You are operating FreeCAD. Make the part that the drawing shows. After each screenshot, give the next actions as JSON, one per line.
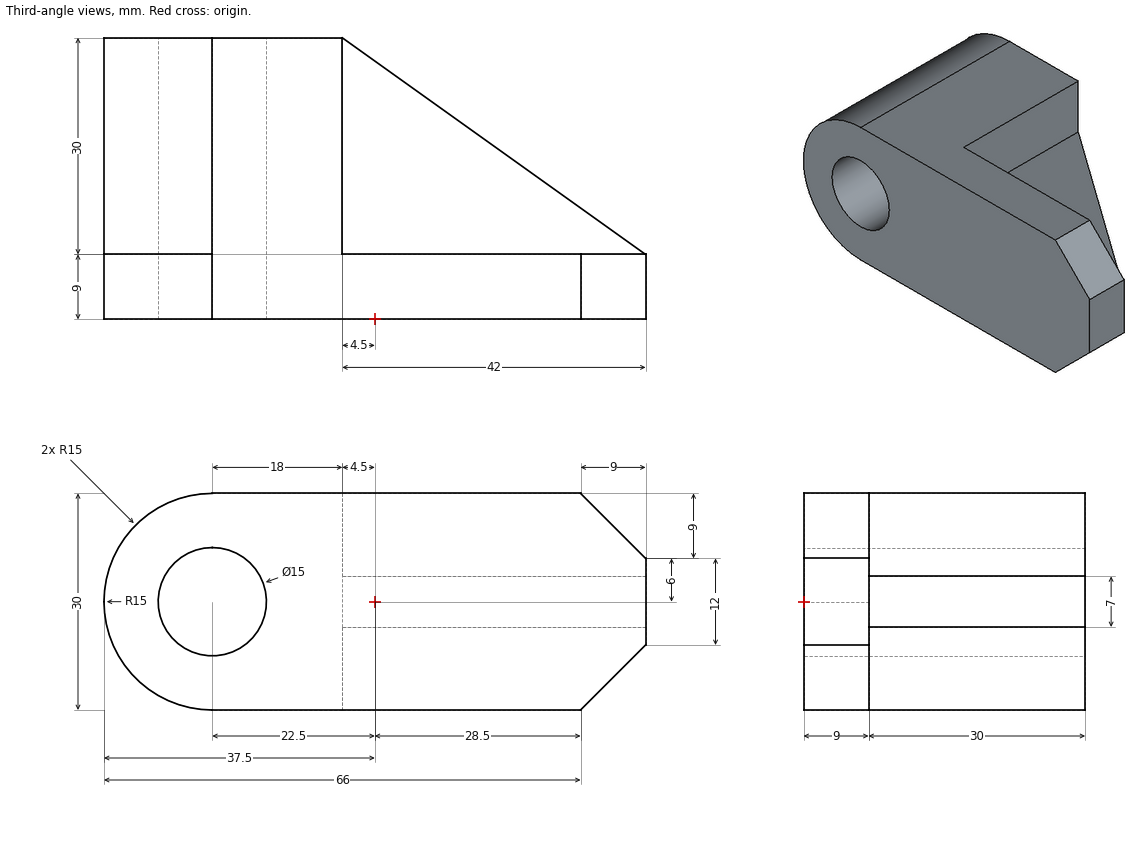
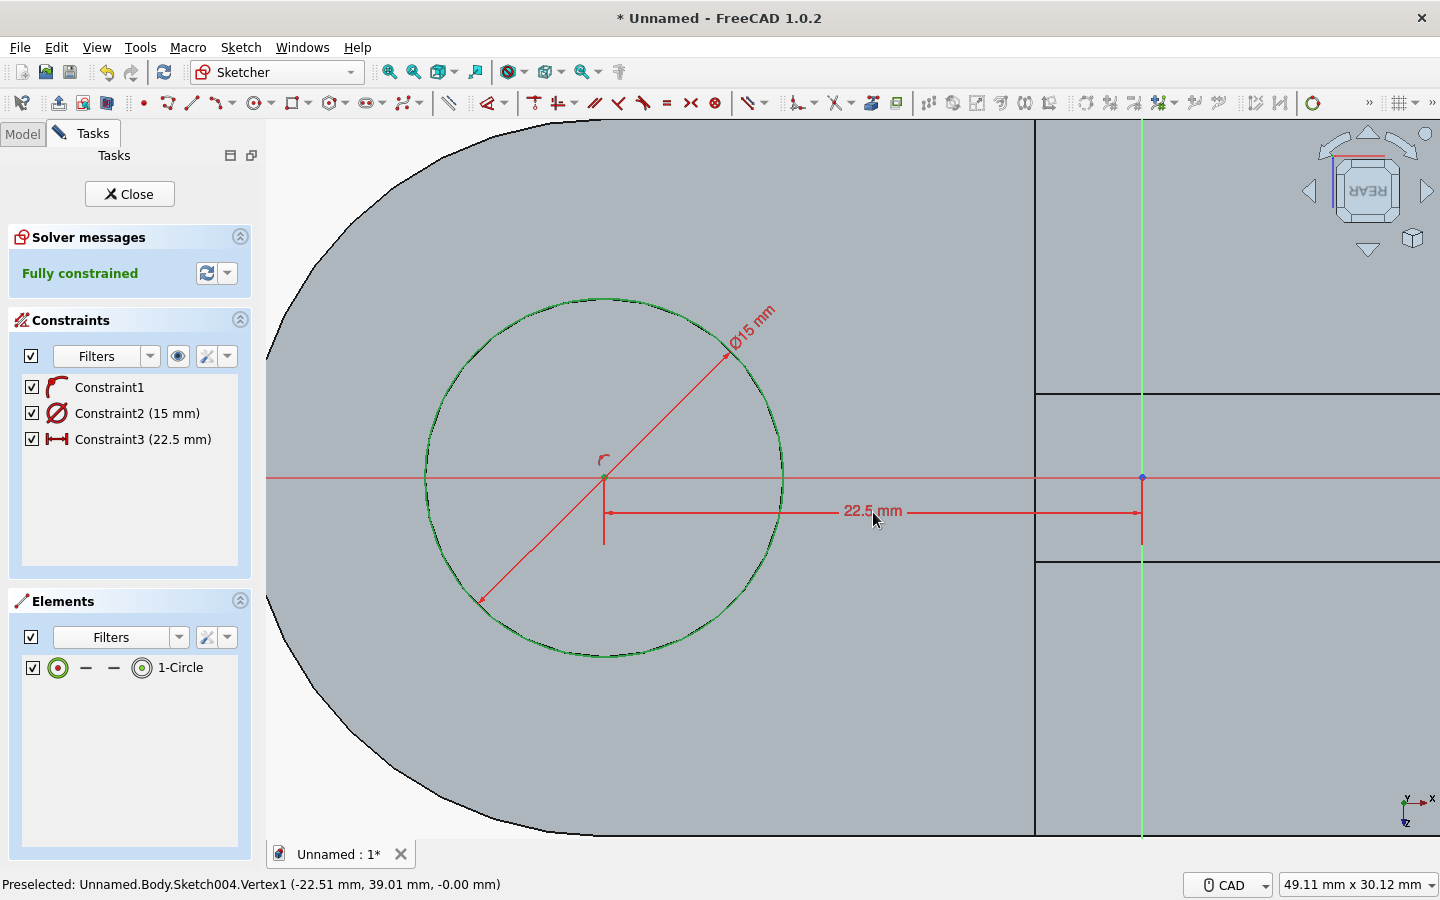
{"action": "left_click", "coordinate": [130, 194]}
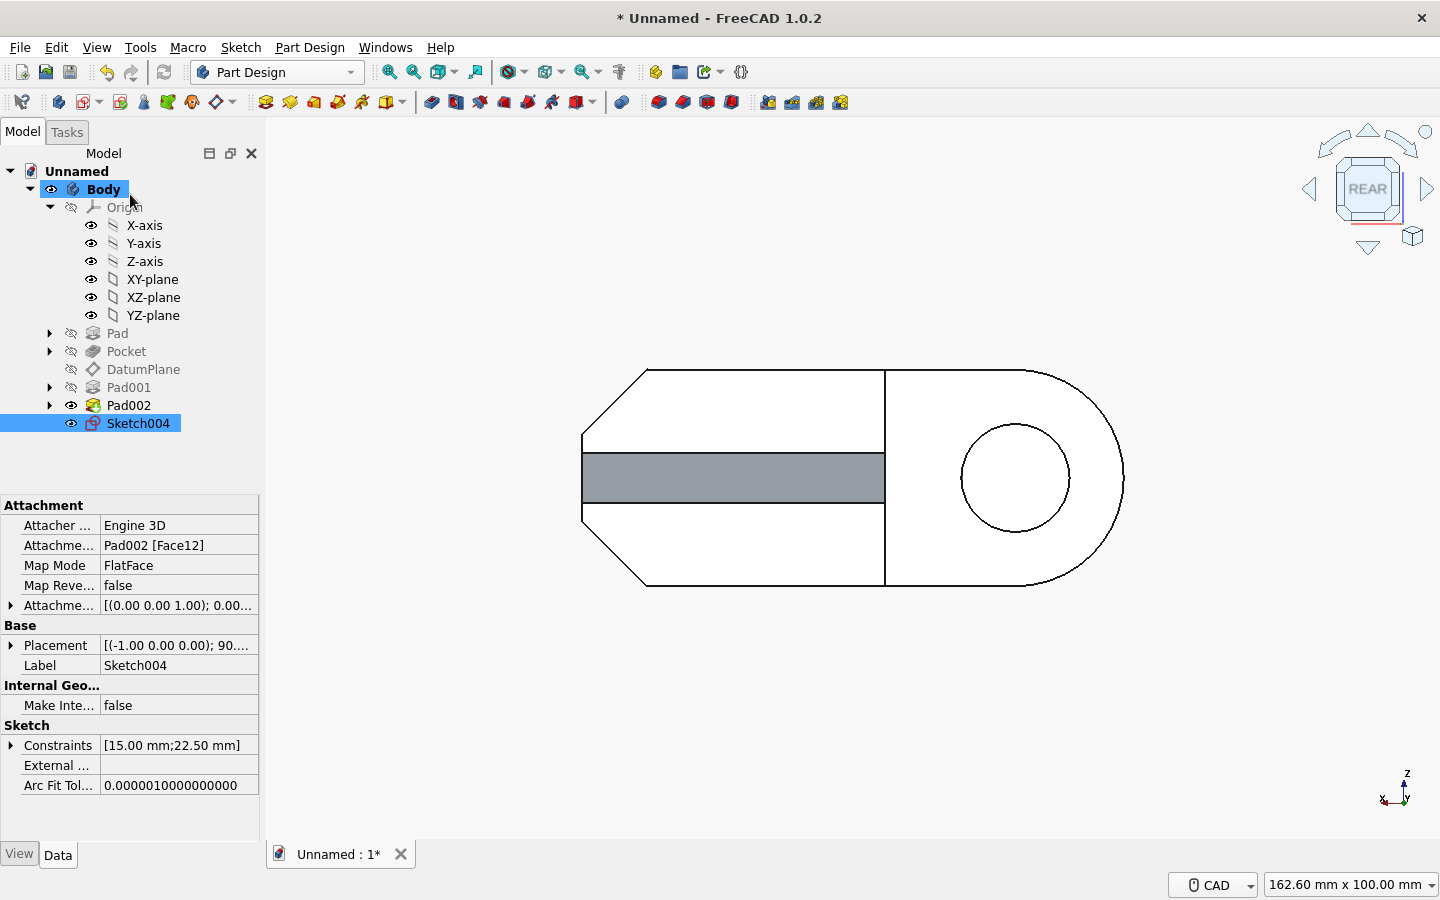
{"action": "left_click", "coordinate": [432, 102]}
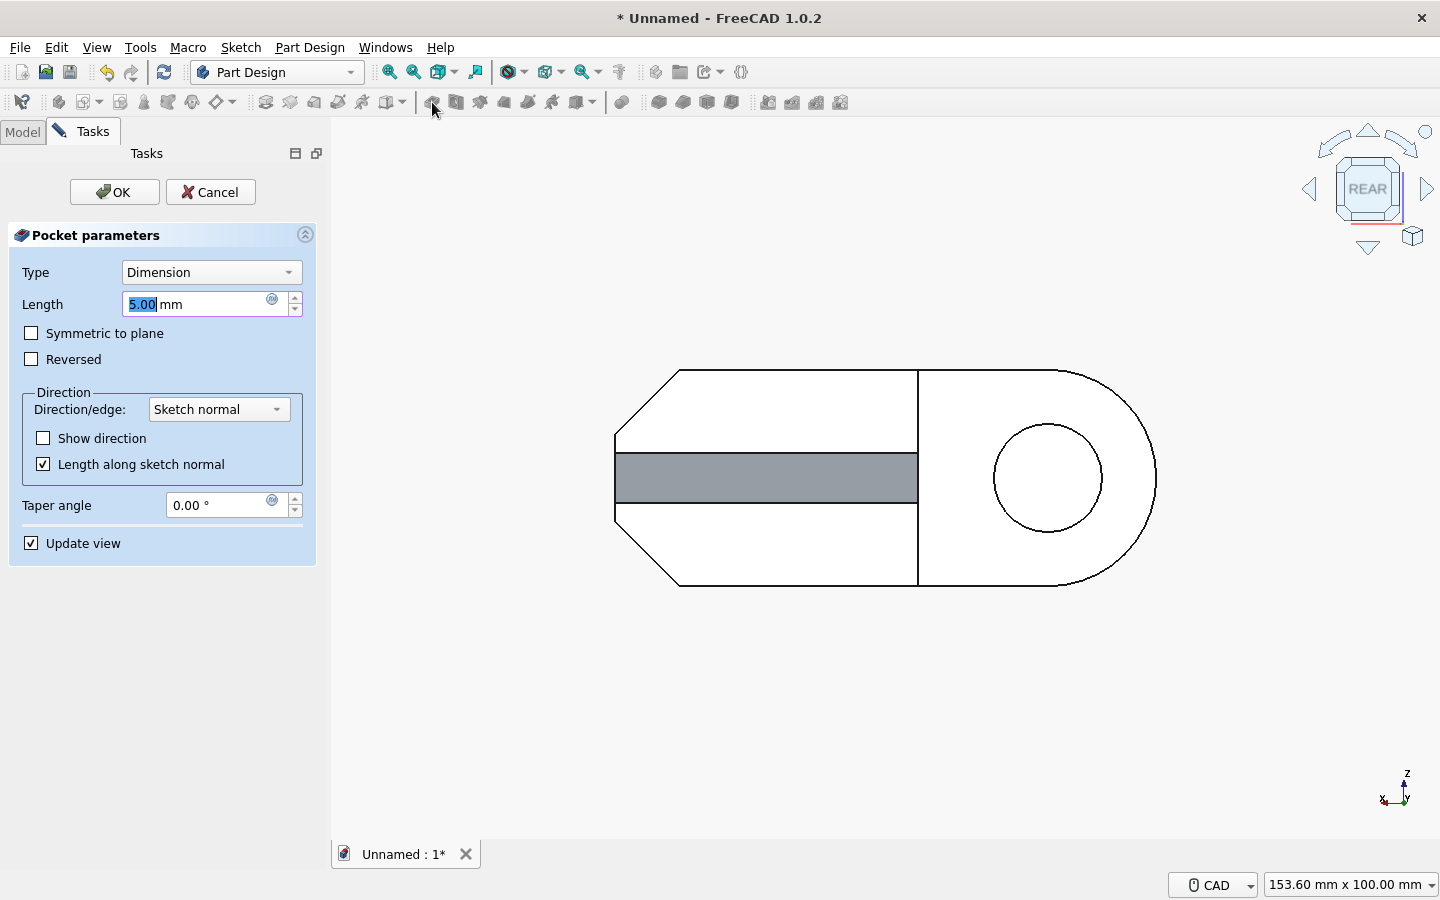
{"action": "left_click", "coordinate": [212, 272]}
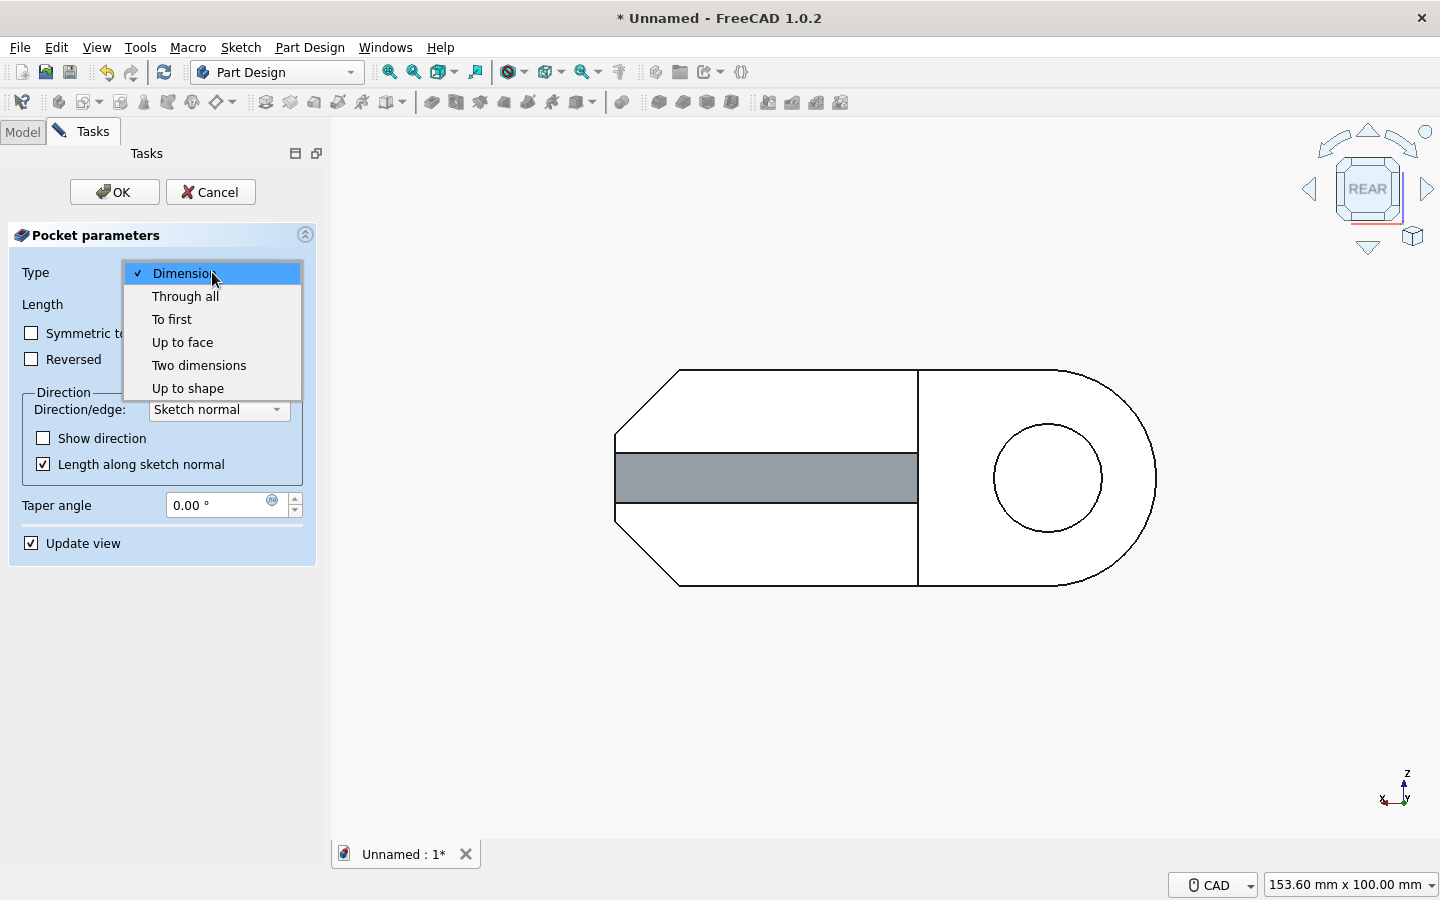
{"action": "left_click", "coordinate": [212, 296]}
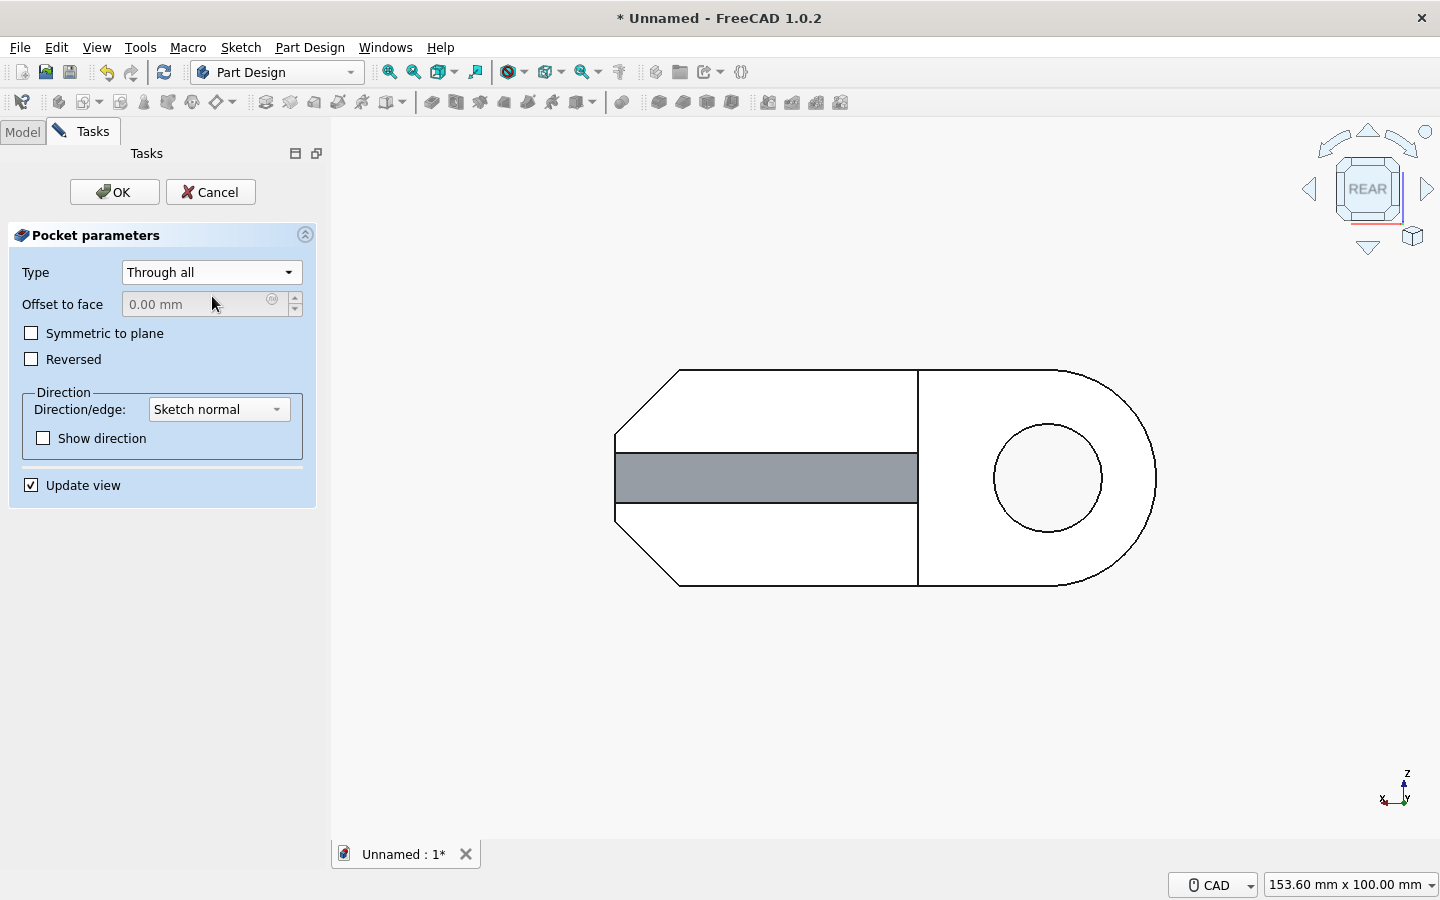
{"action": "left_click", "coordinate": [115, 192]}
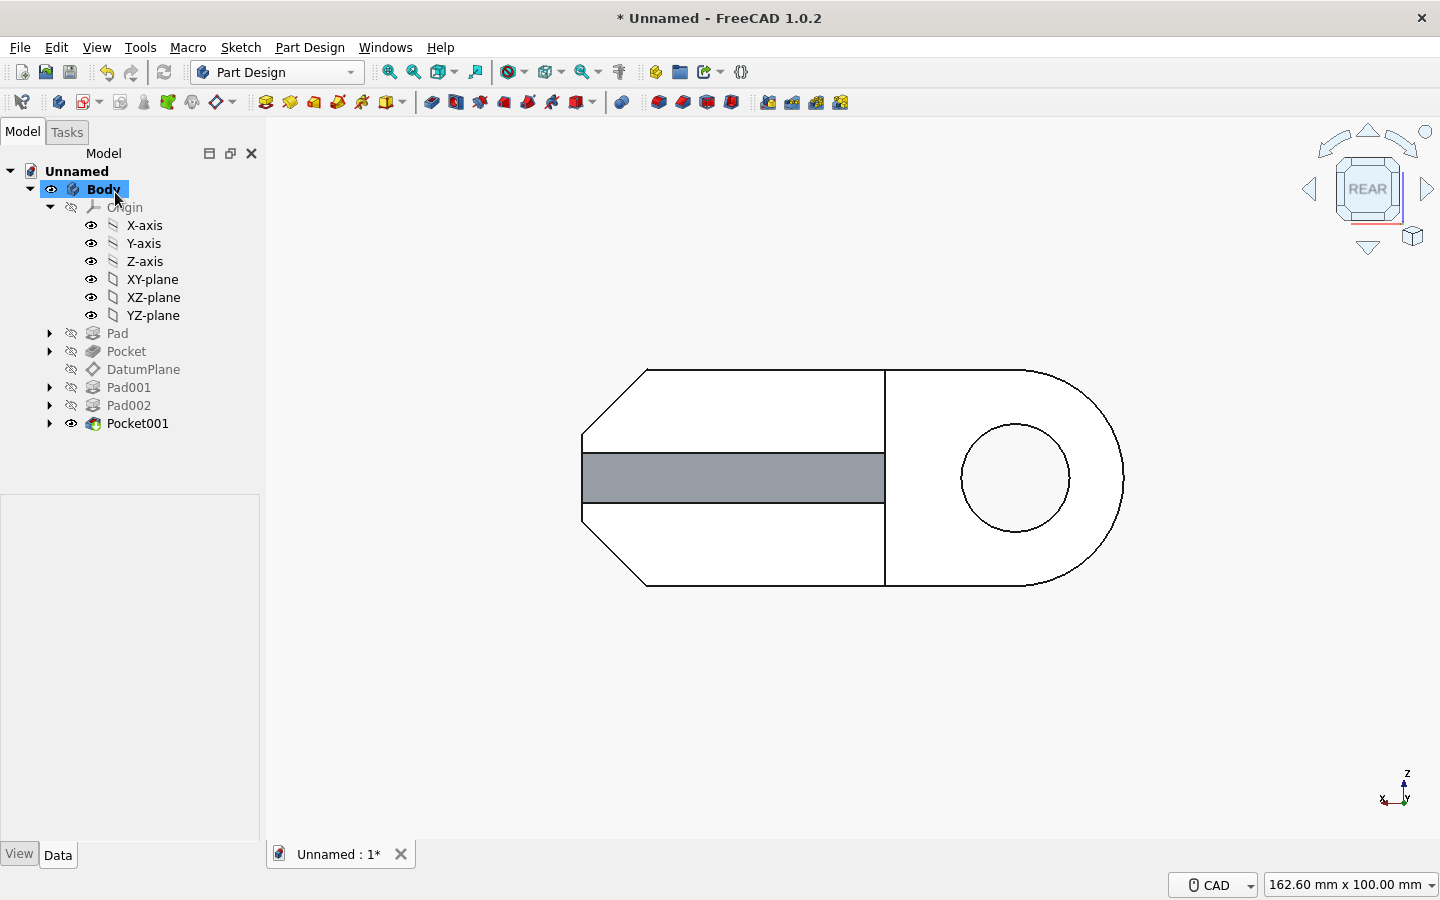
{"action": "key", "text": "0"}